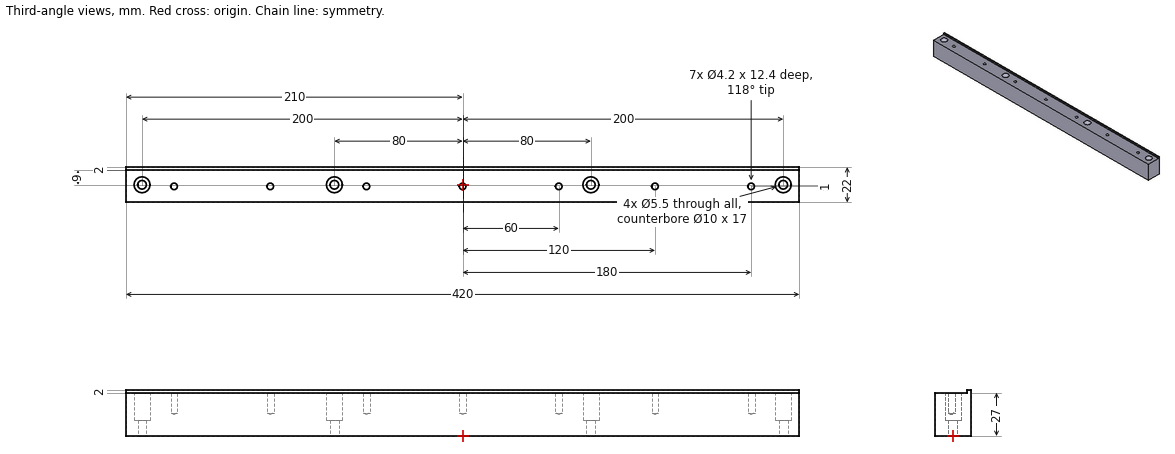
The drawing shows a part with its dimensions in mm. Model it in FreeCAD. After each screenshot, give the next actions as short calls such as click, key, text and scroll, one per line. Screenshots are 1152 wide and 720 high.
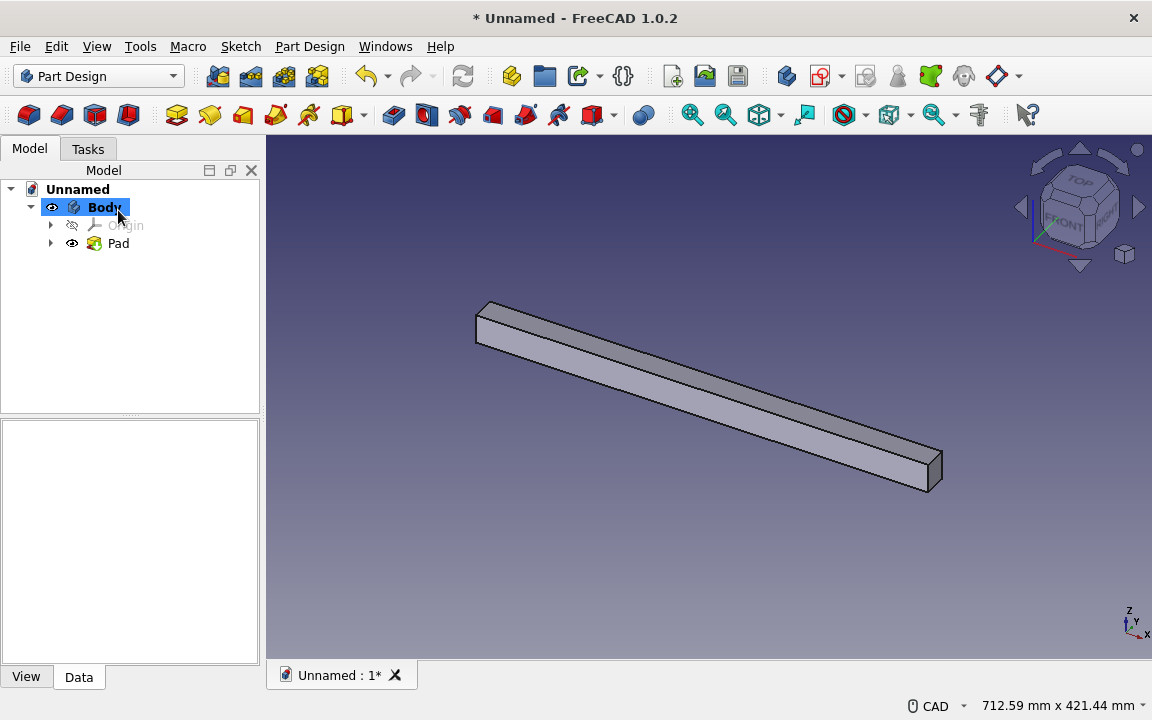
click(903, 446)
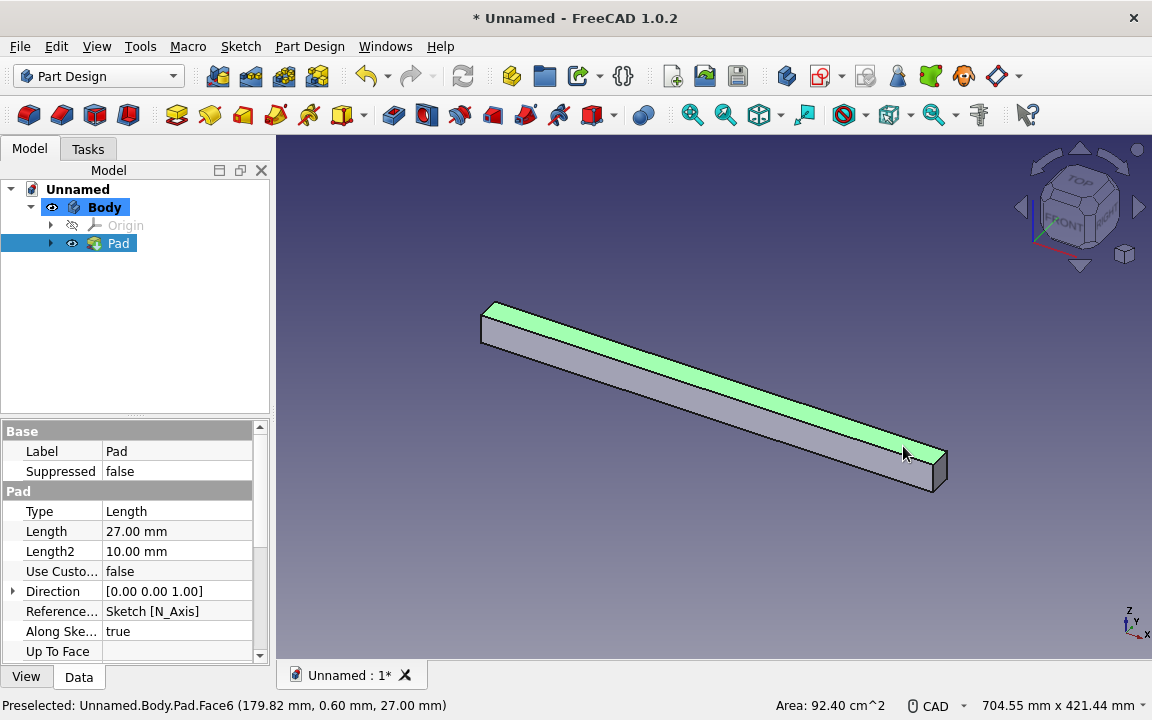
click(820, 76)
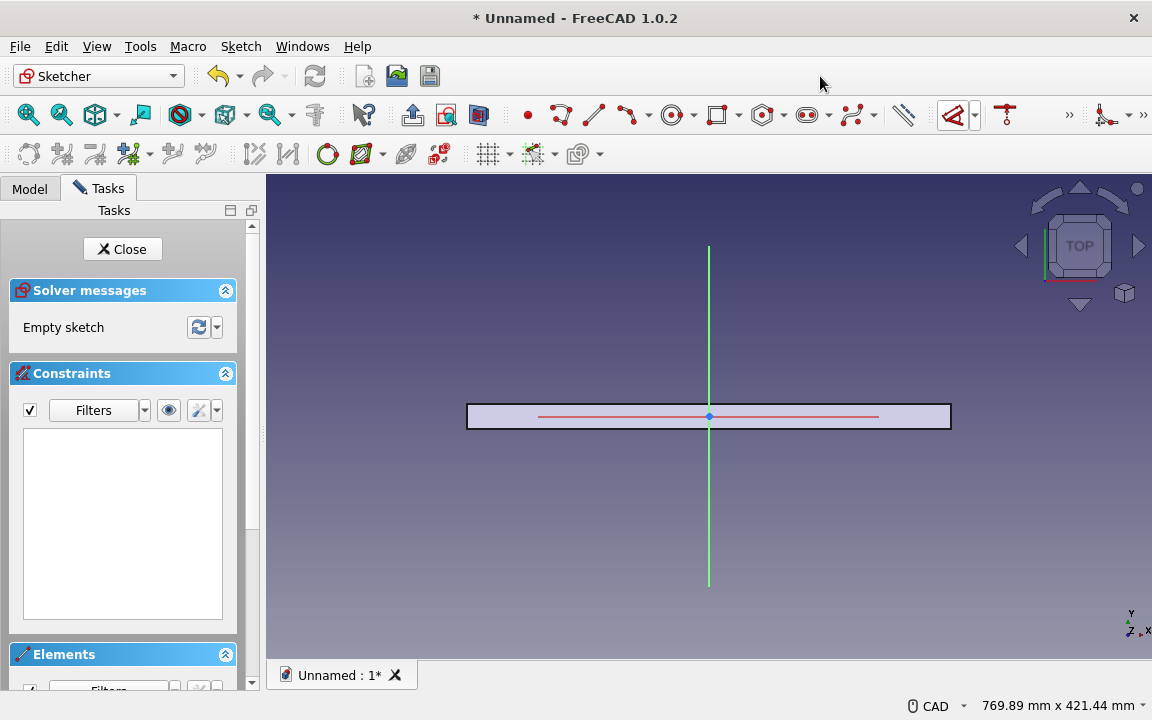
key(g)
key(r)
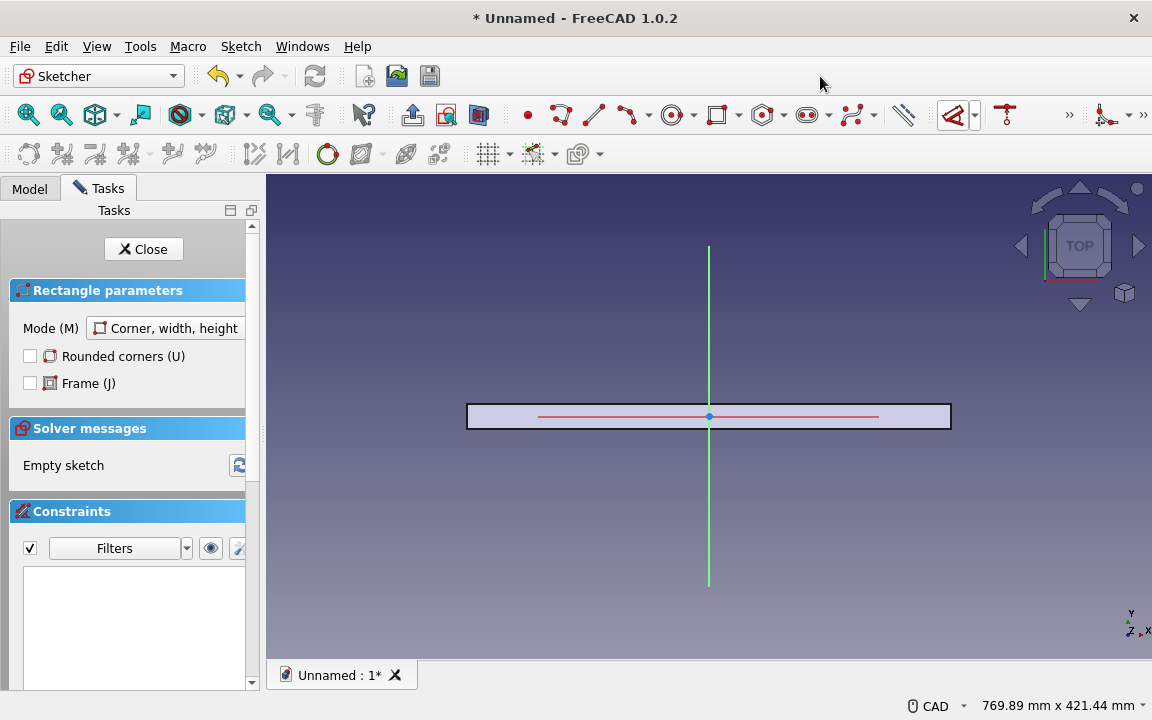
scroll(467, 404, up, 10)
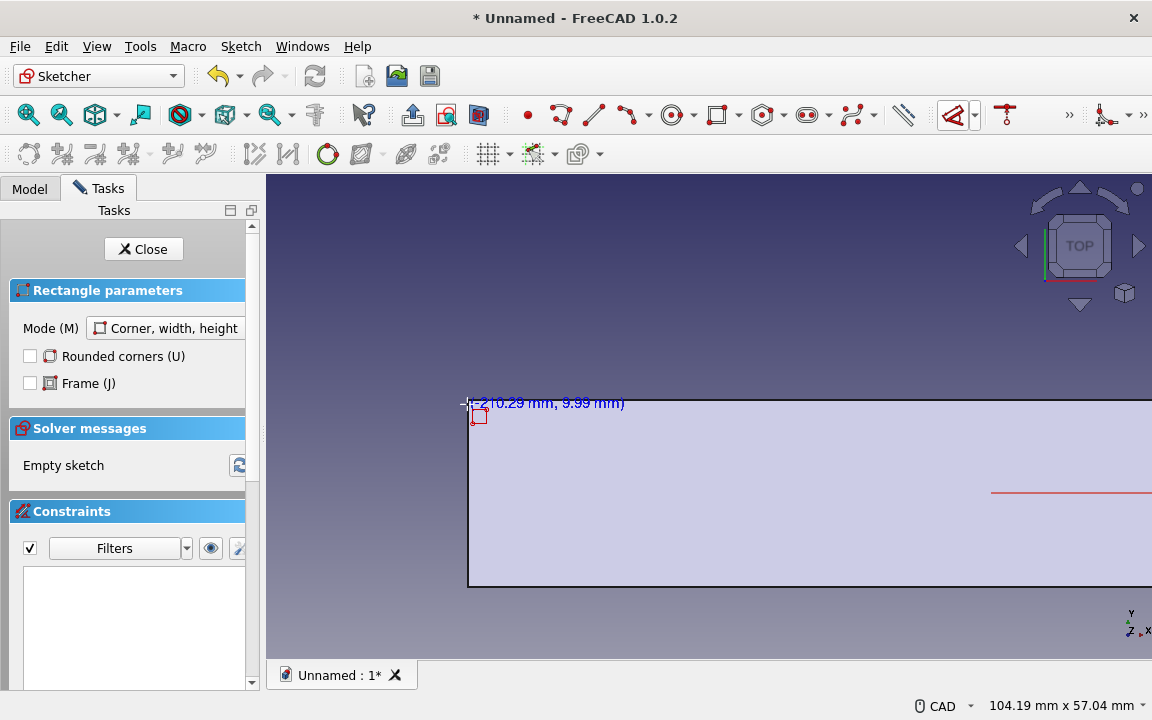
scroll(388, 412, down, 10)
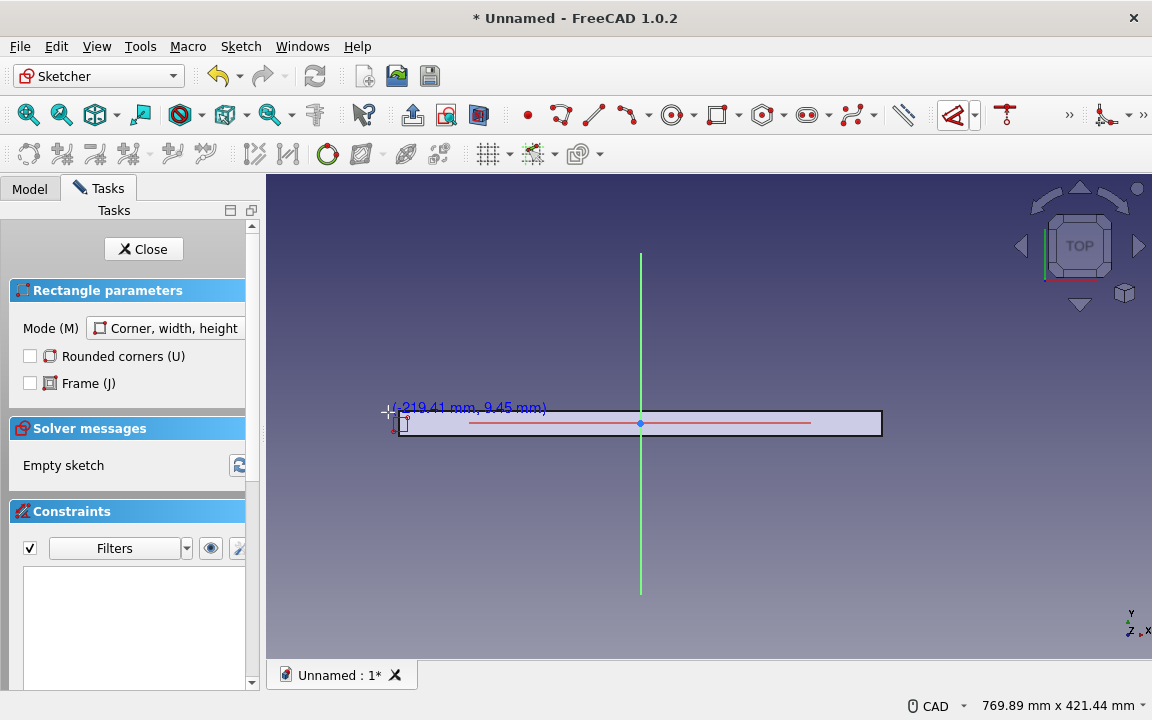
scroll(399, 411, up, 2)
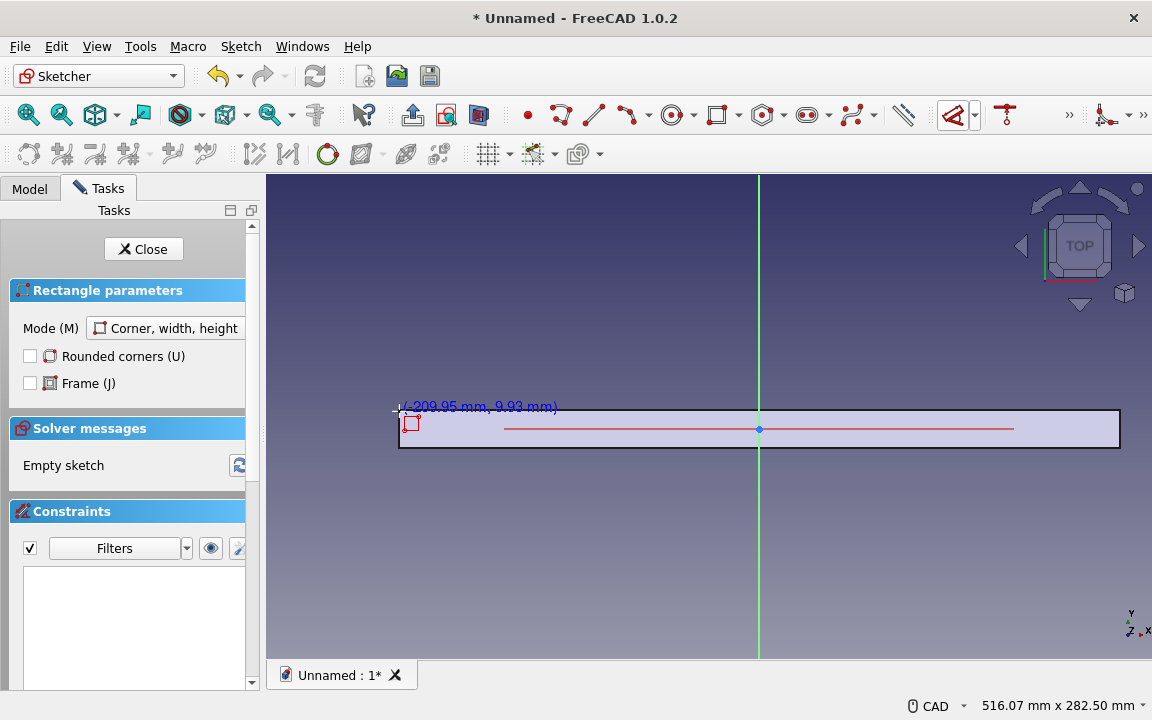
click(399, 410)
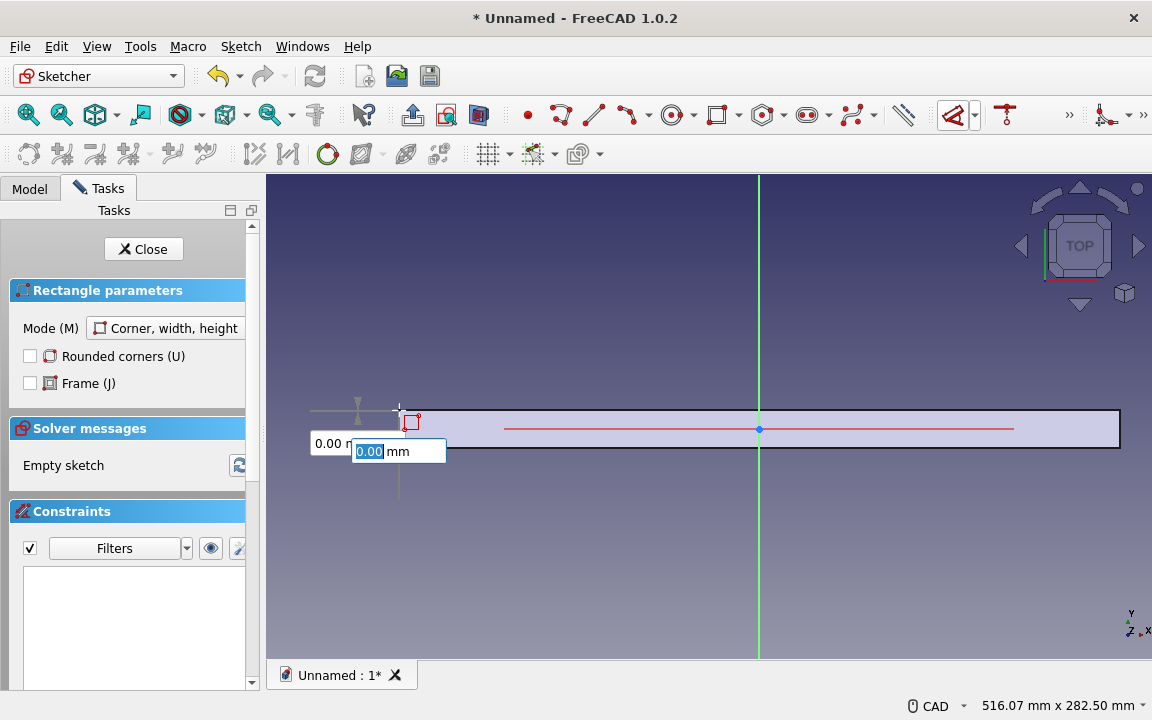
scroll(399, 410, down, 2)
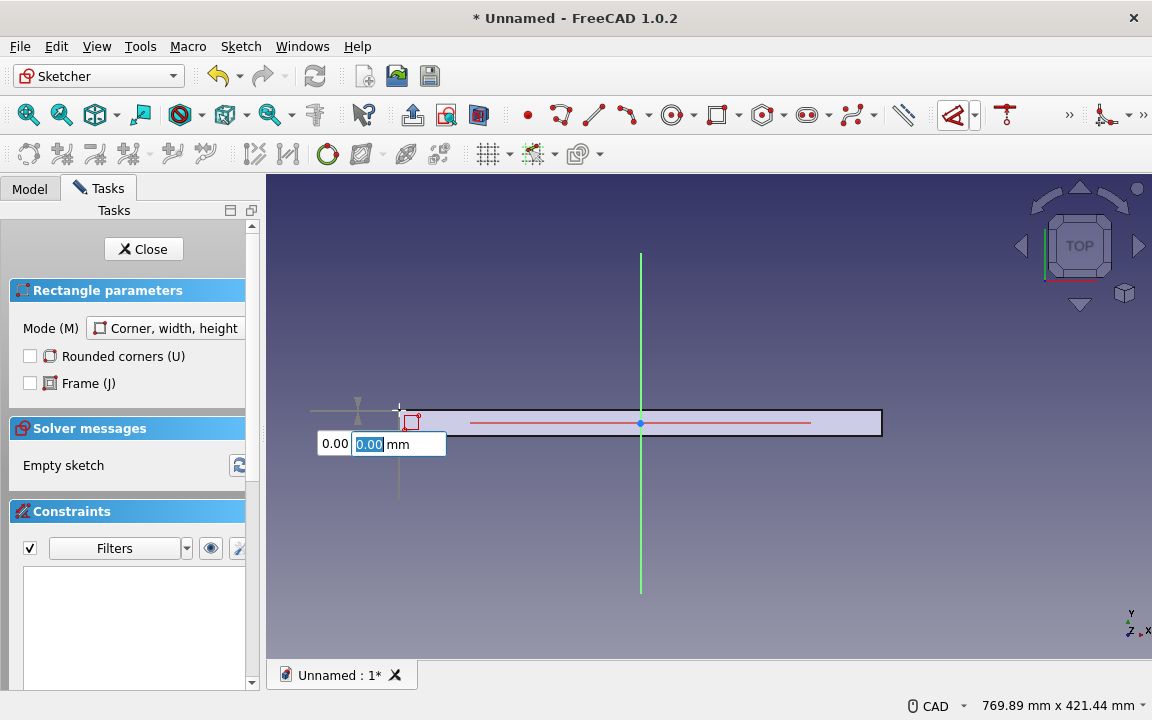
scroll(882, 413, up, 3)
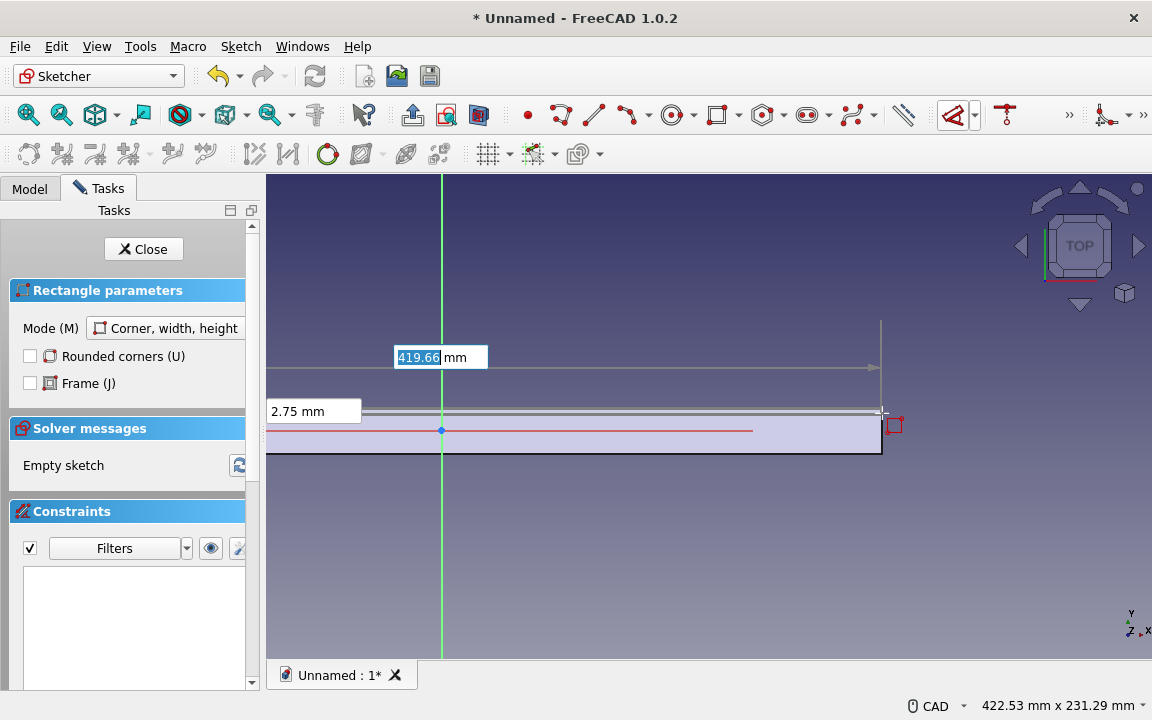
click(882, 412)
key(Escape)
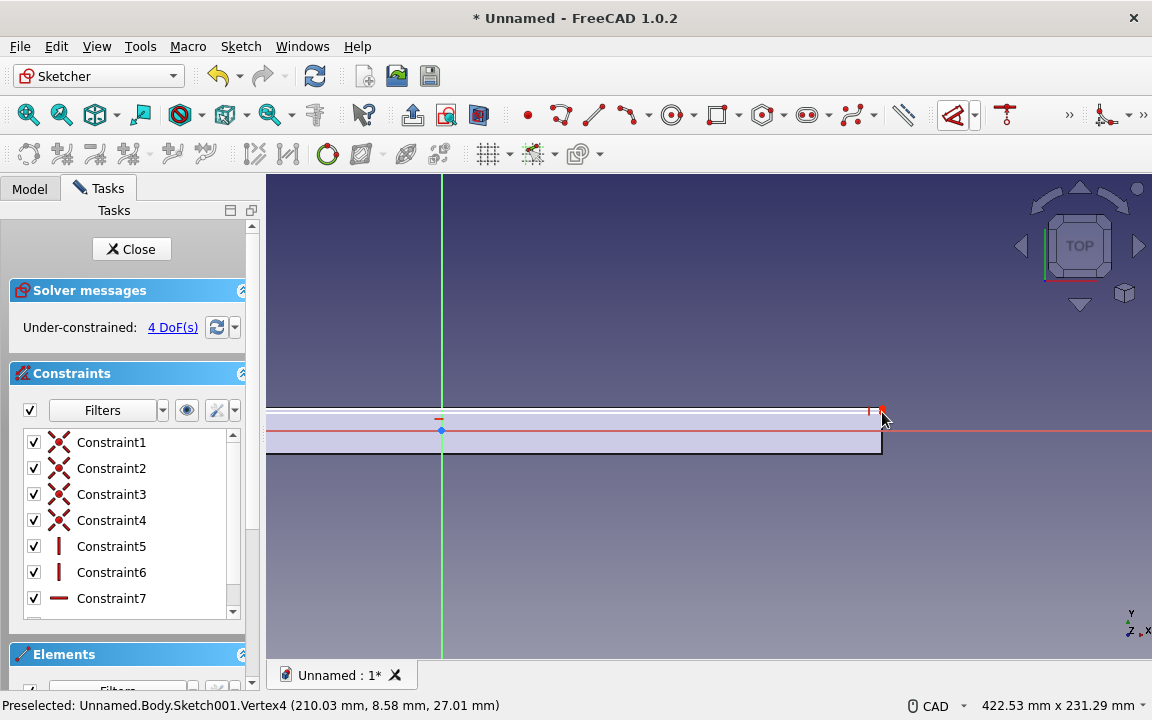
key(d)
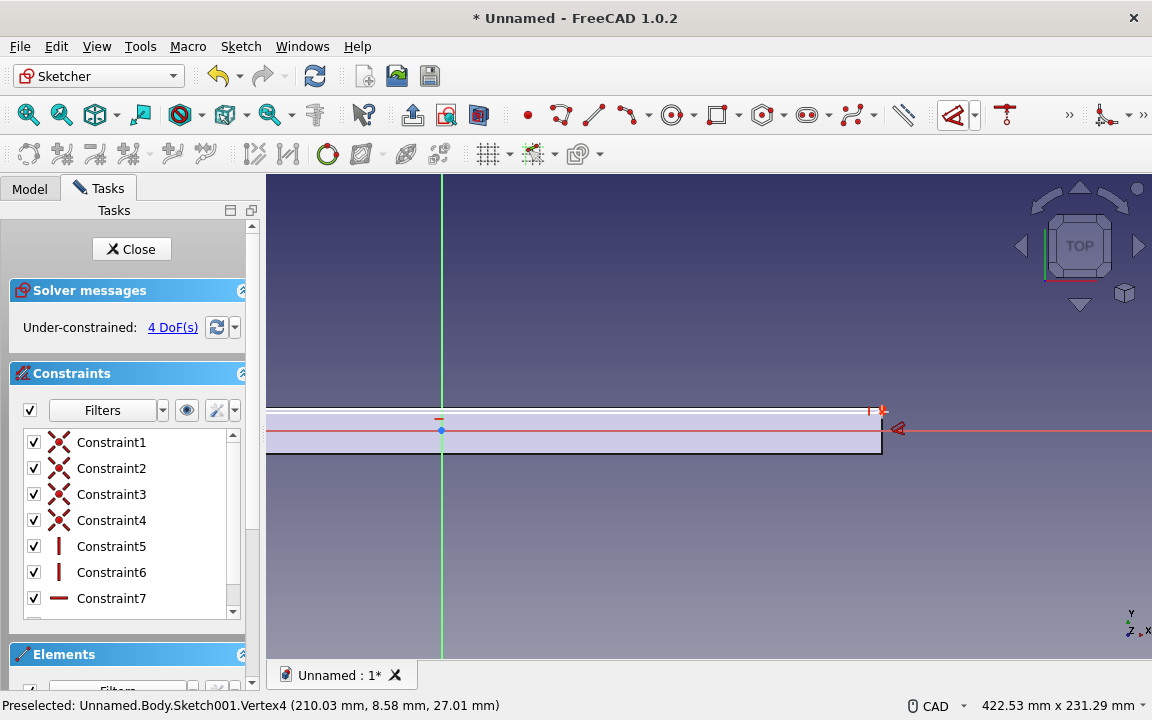
scroll(882, 413, down, 3)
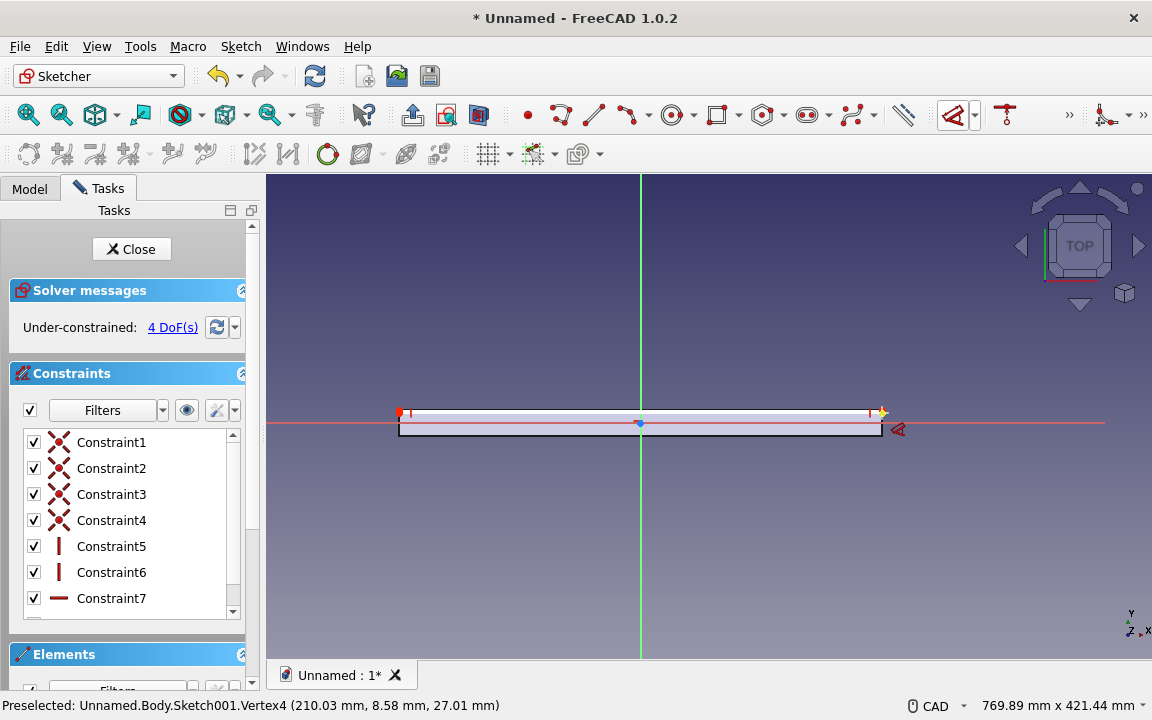
scroll(399, 412, up, 15)